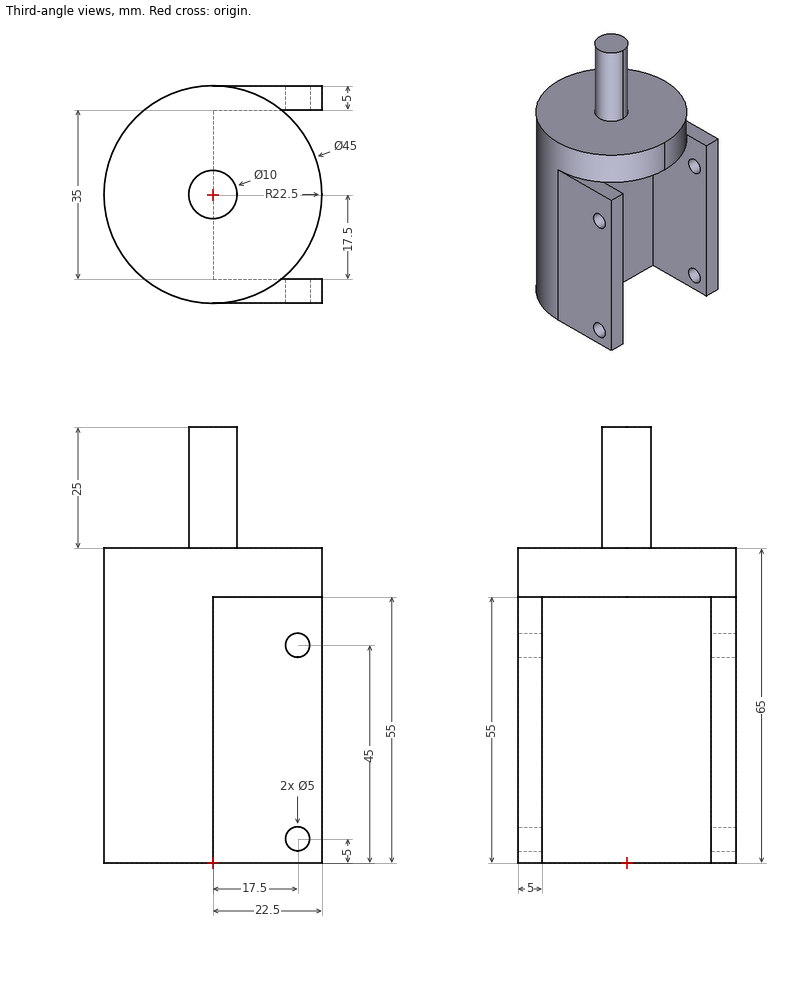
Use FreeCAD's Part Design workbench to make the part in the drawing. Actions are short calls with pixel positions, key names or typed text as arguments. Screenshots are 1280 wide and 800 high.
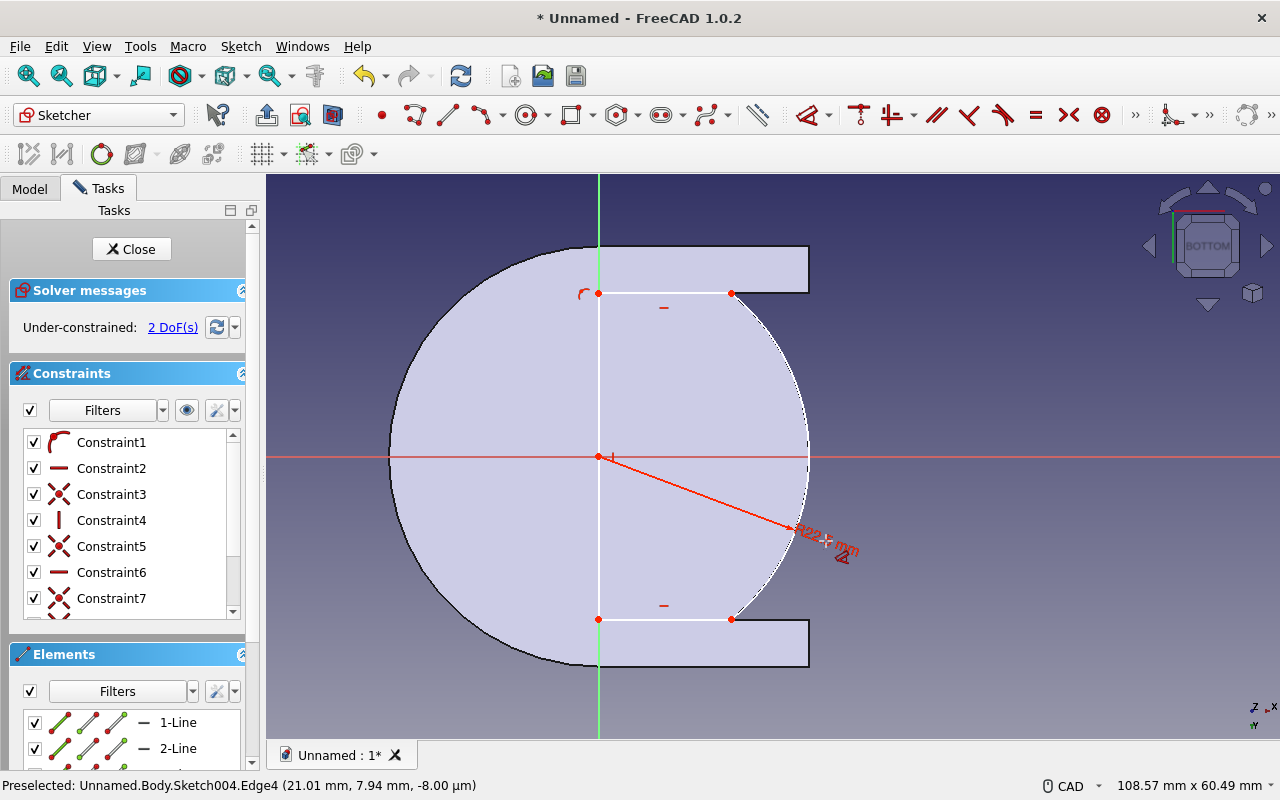
click(599, 391)
click(565, 381)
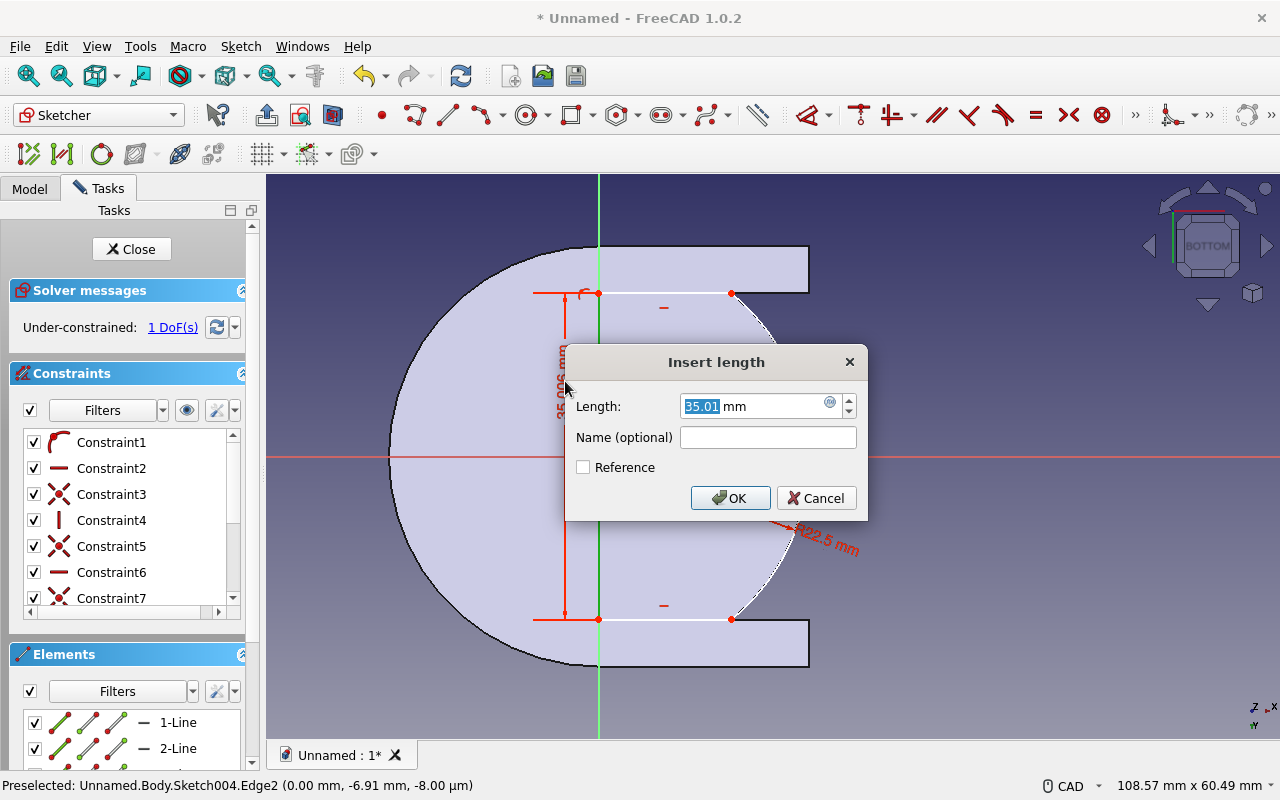
text(35)
key(Return)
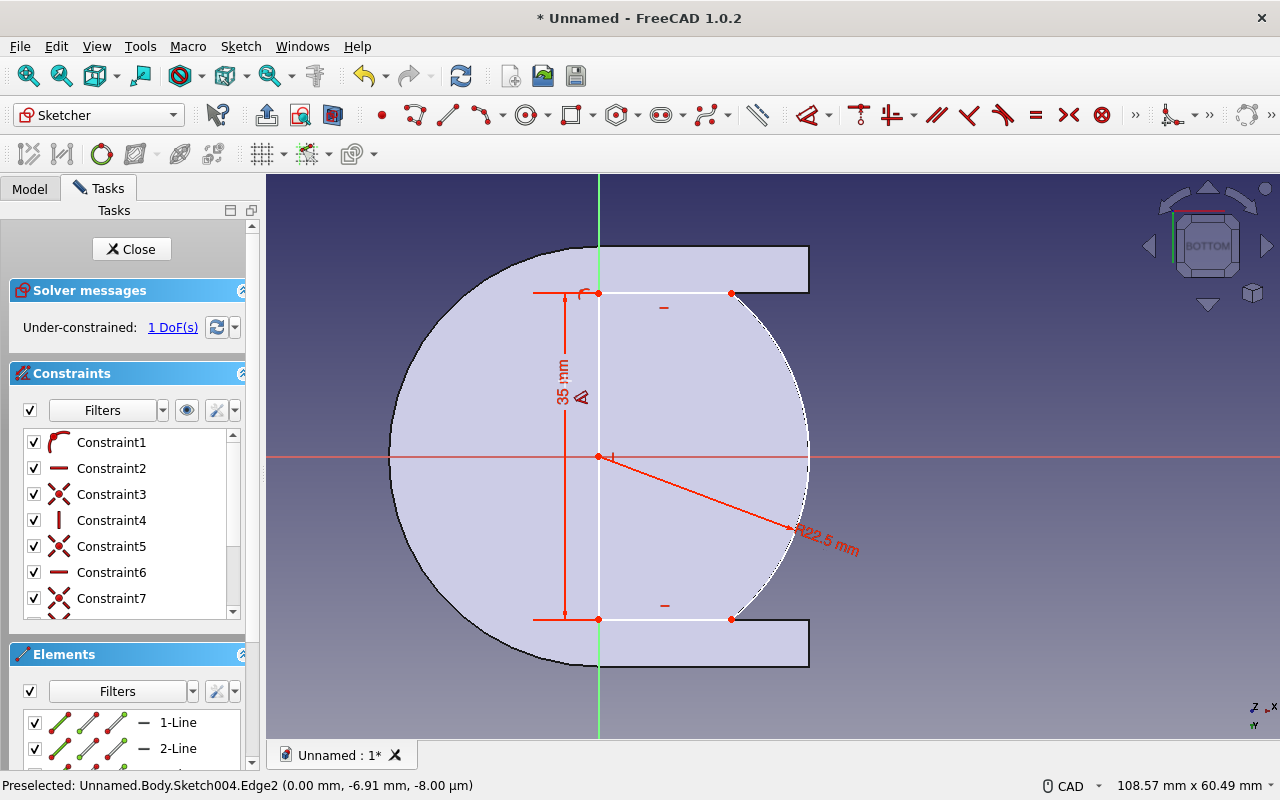
click(731, 293)
click(565, 337)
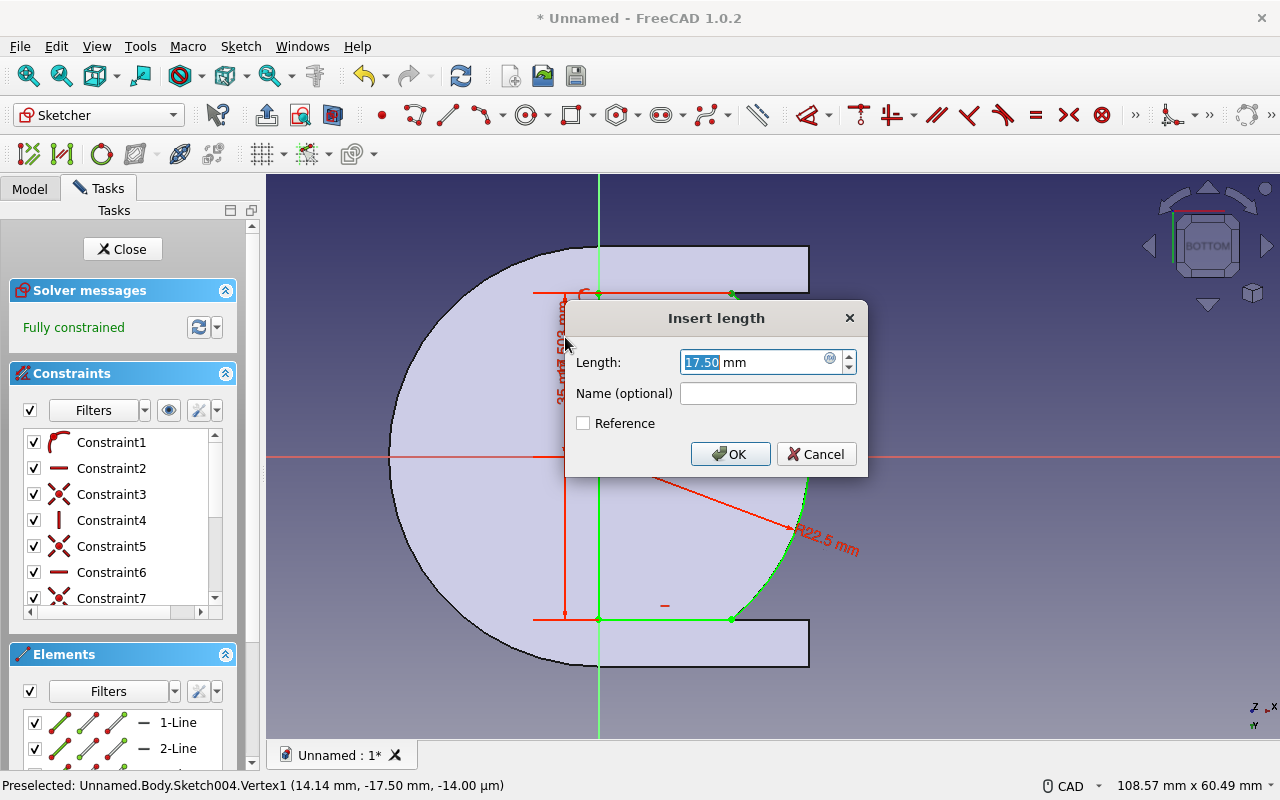
text(17.5)
key(Return)
key(Escape)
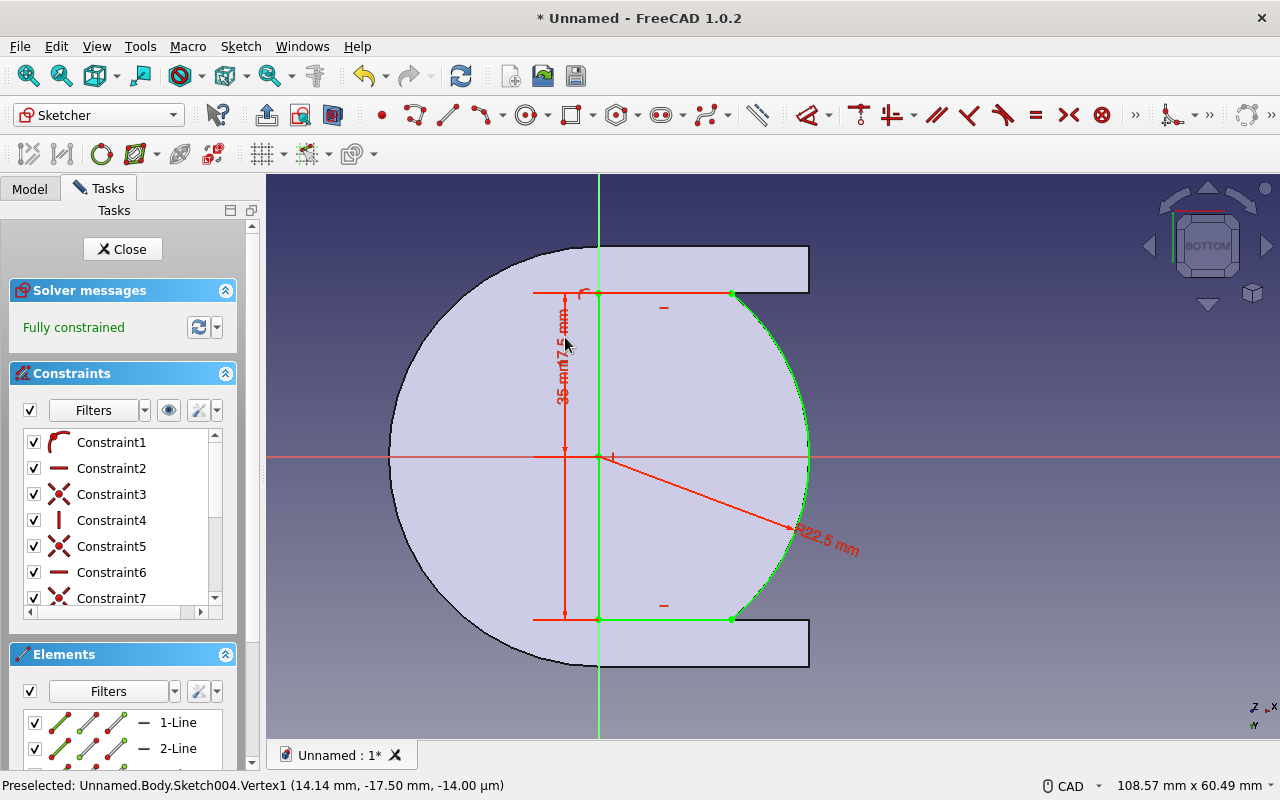
click(123, 249)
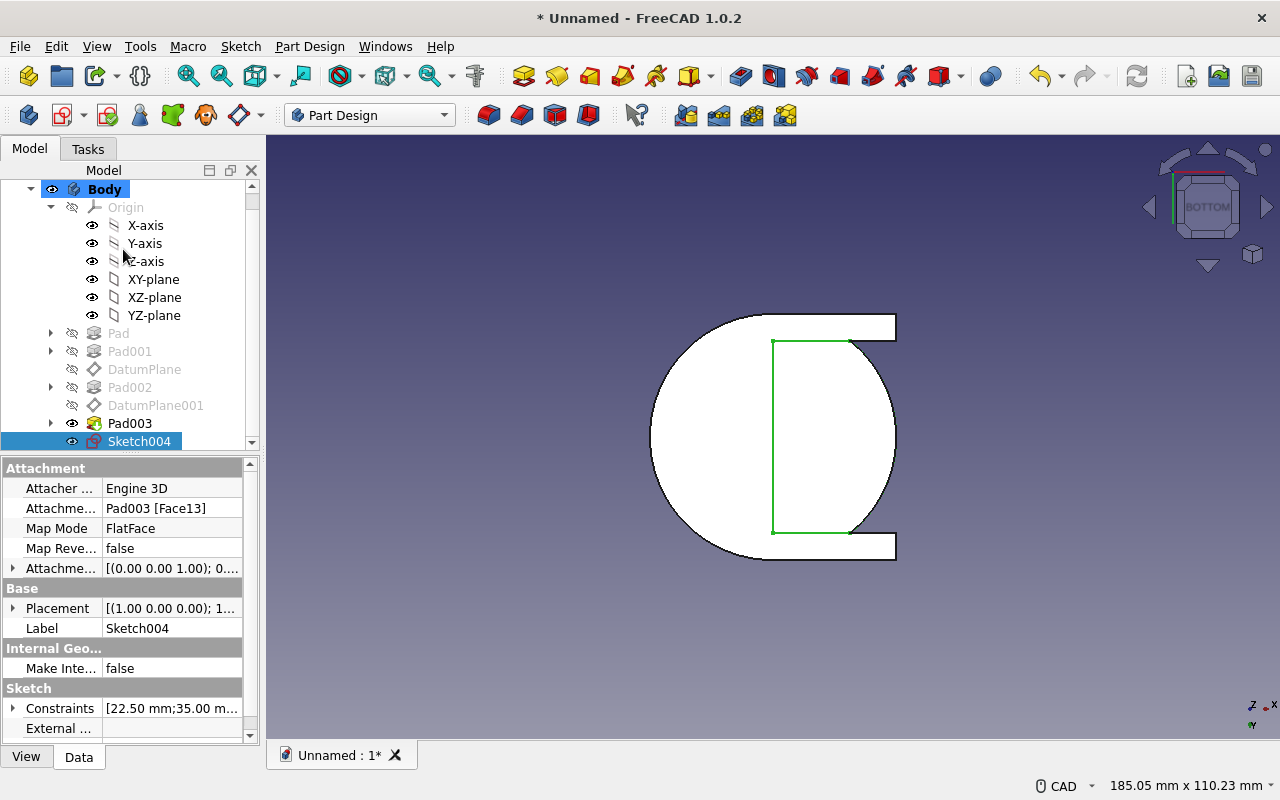
click(741, 76)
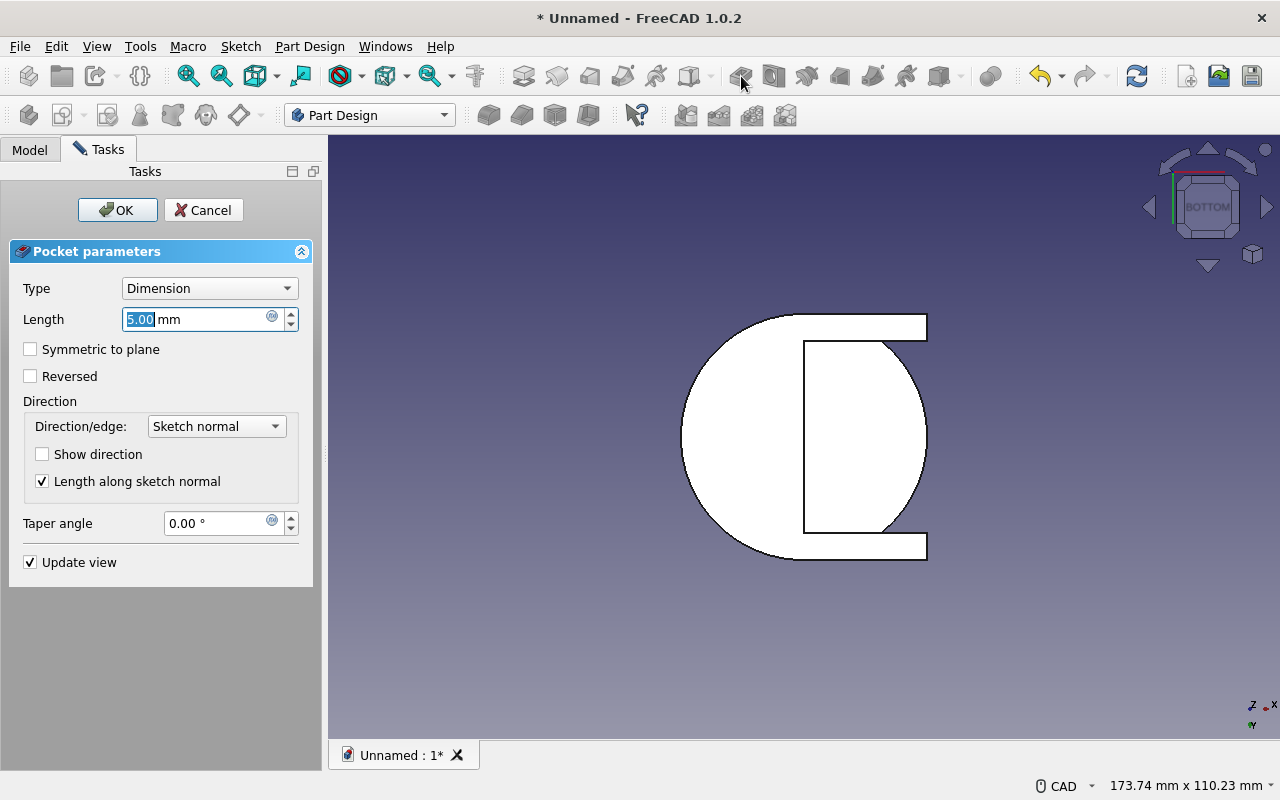
text(55)
key(Tab)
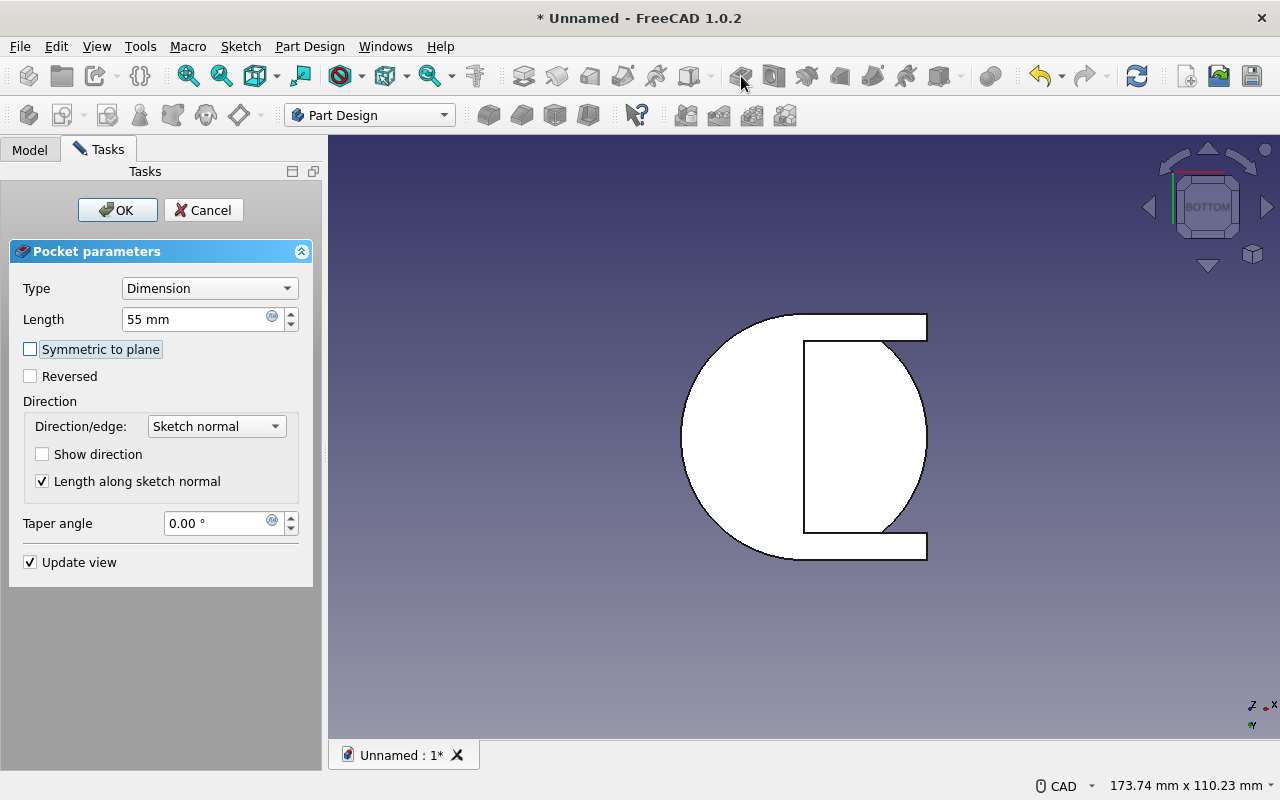
click(118, 210)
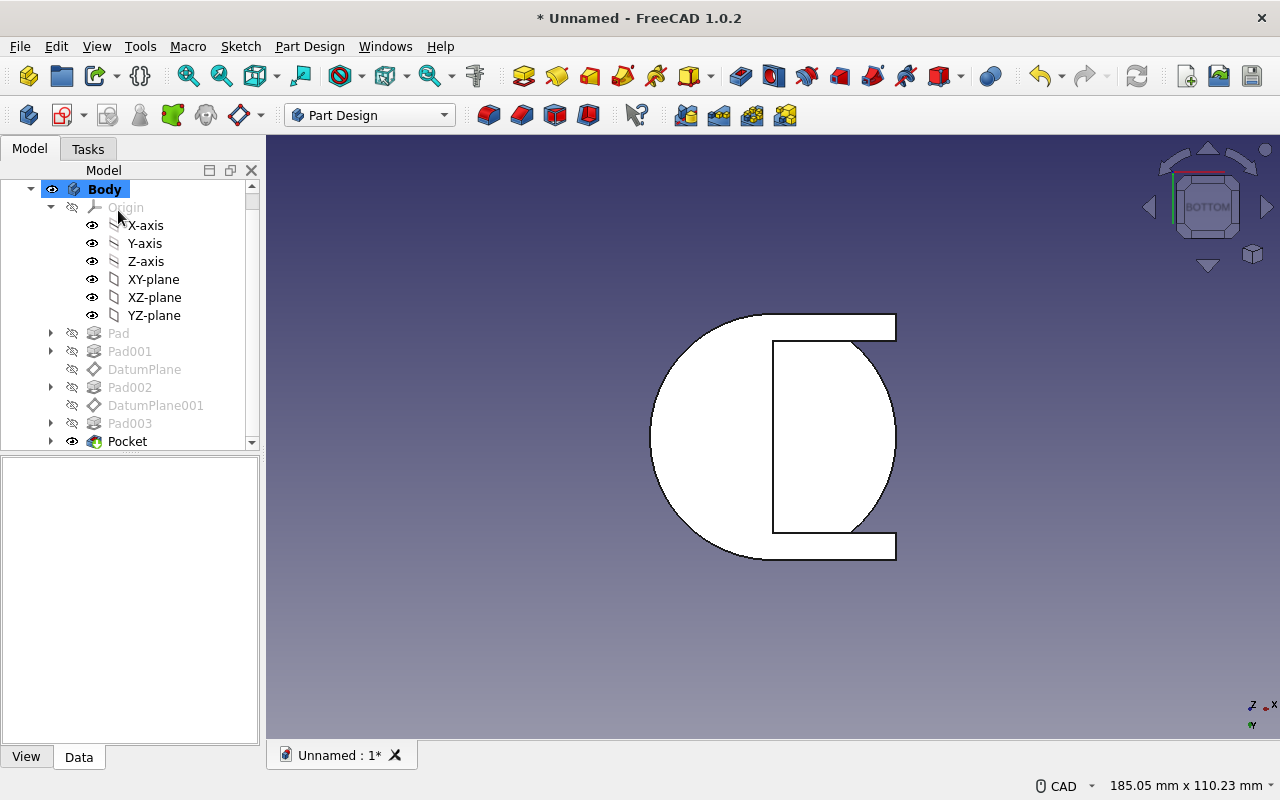
click(189, 76)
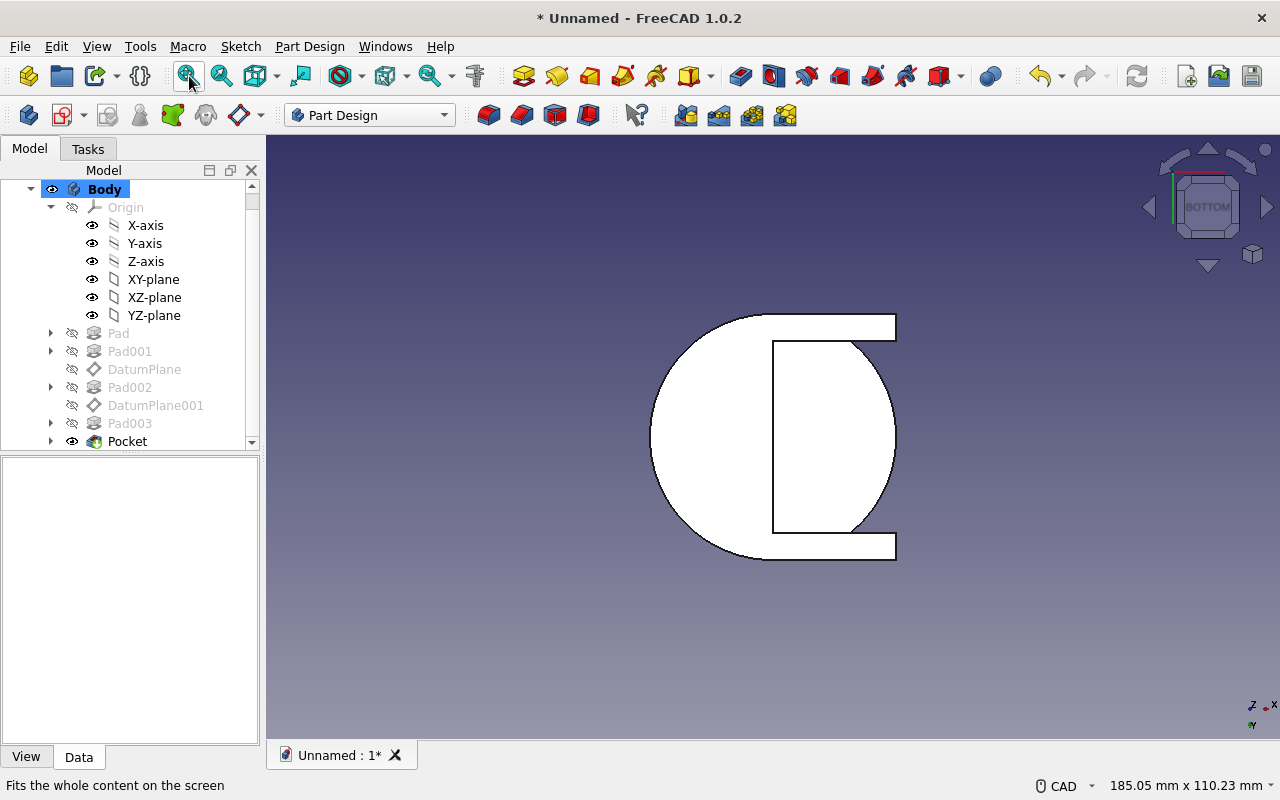
key(0)